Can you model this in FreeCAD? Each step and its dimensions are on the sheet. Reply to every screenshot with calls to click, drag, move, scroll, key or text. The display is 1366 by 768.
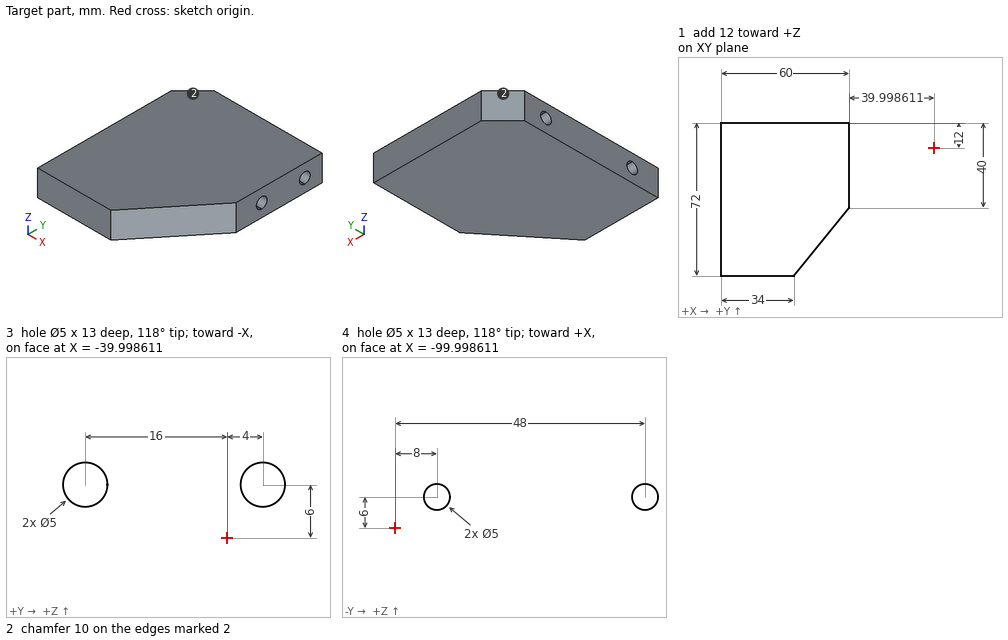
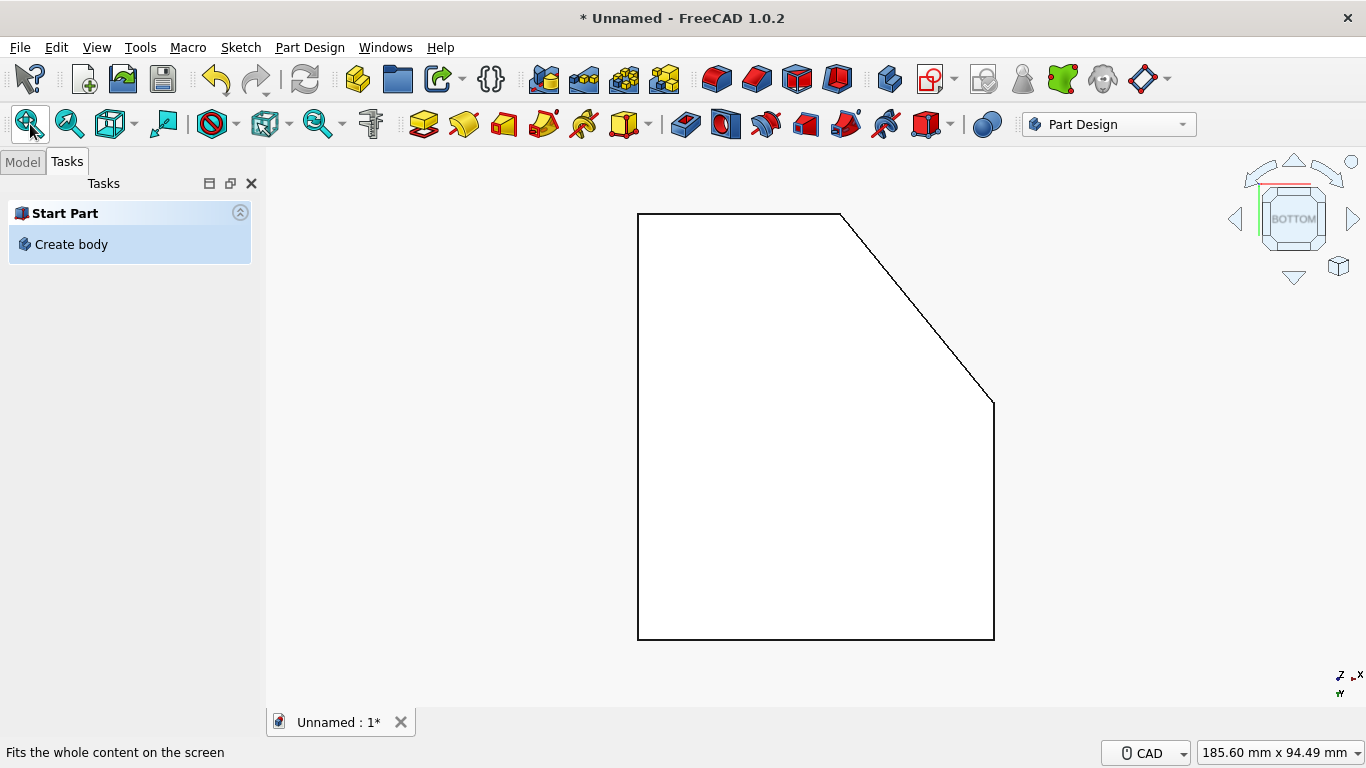
key(4)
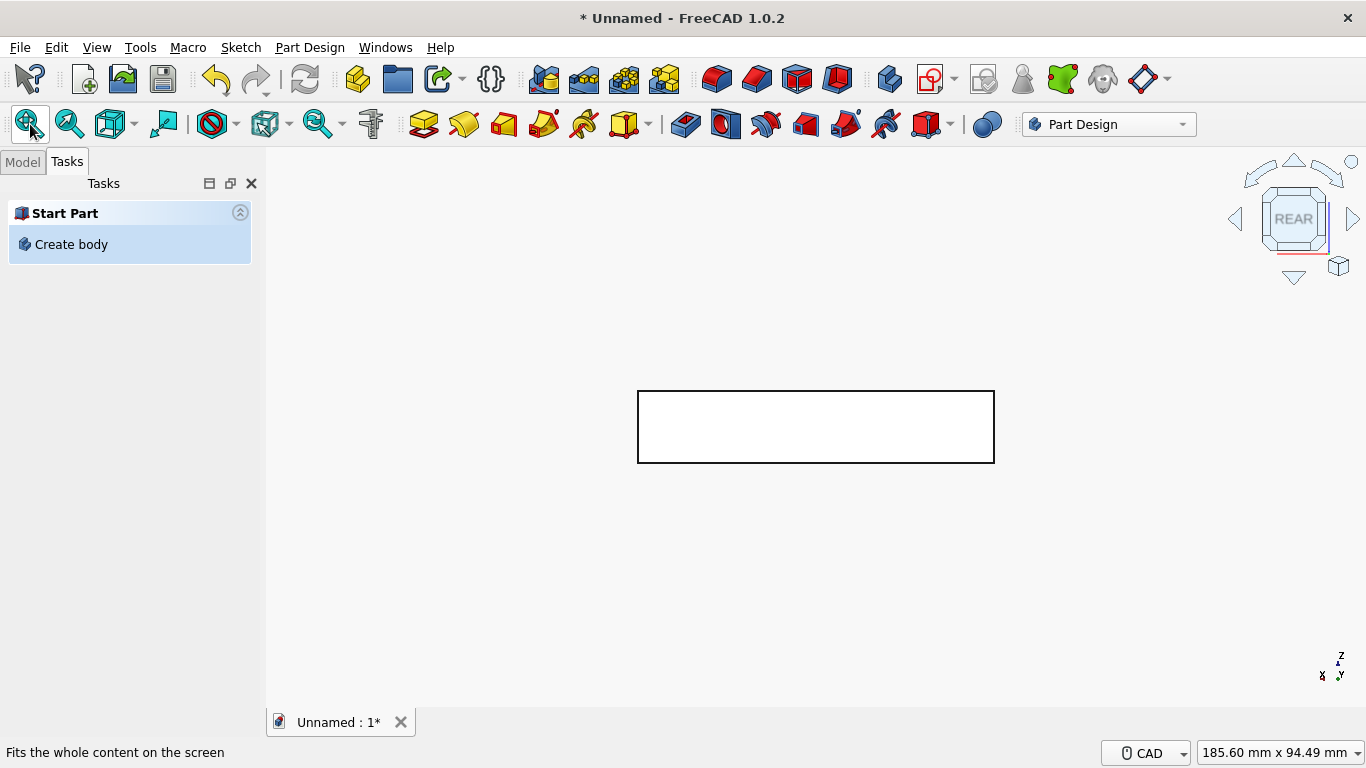
key(v)
key(f)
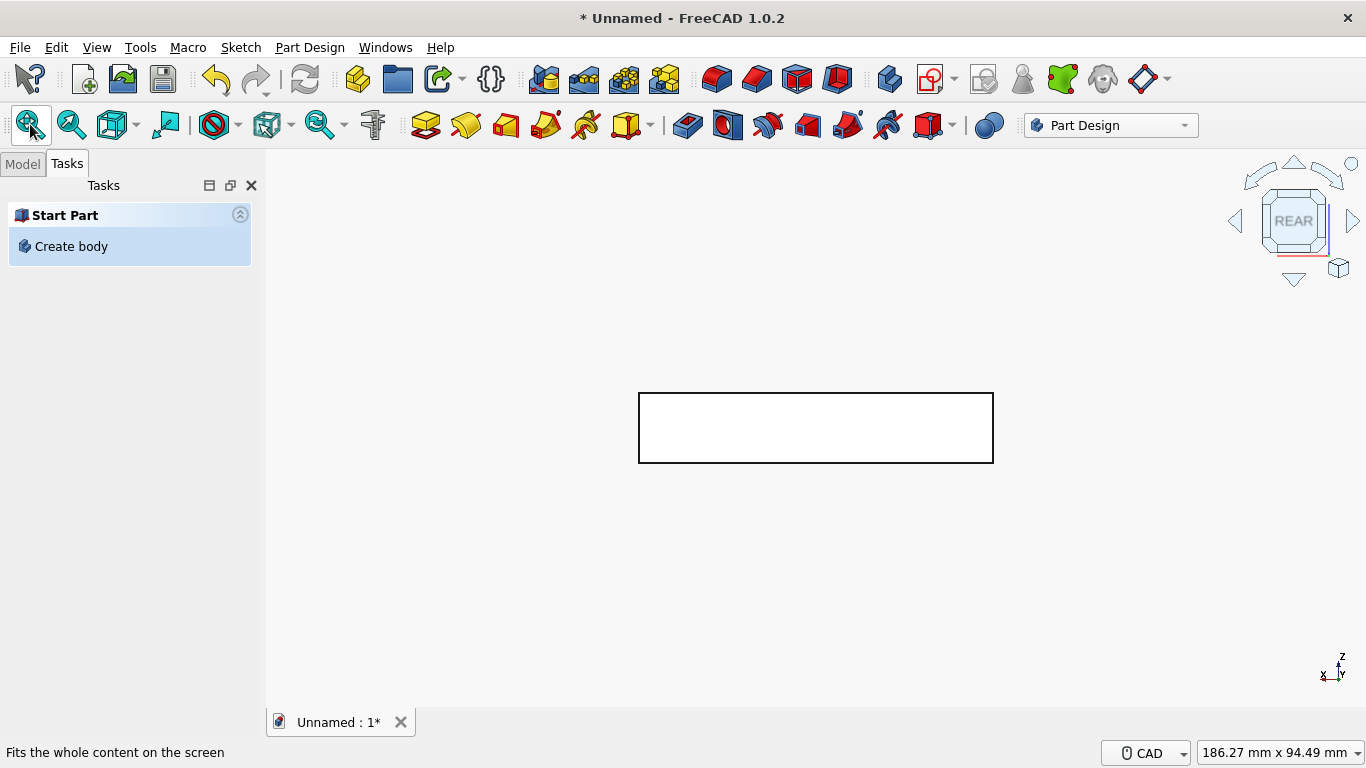
click(993, 427)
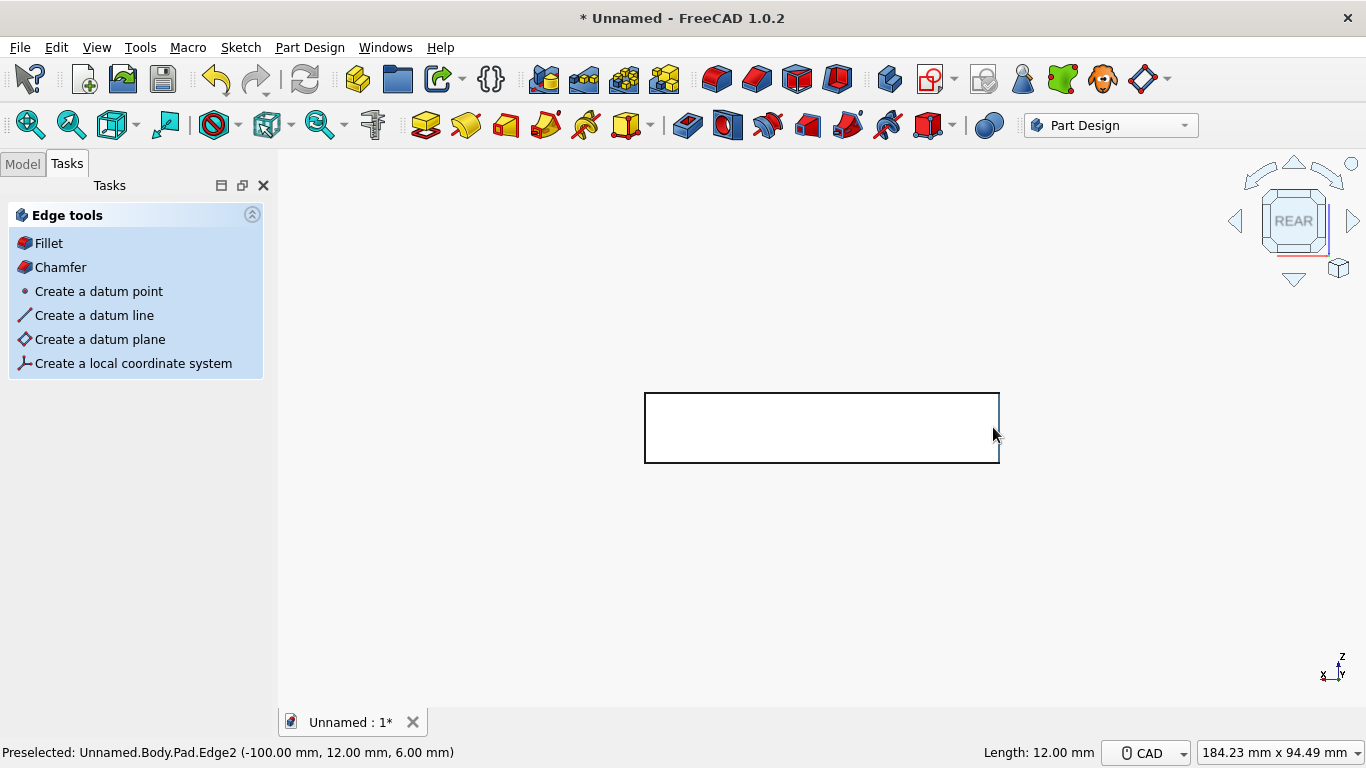
click(758, 80)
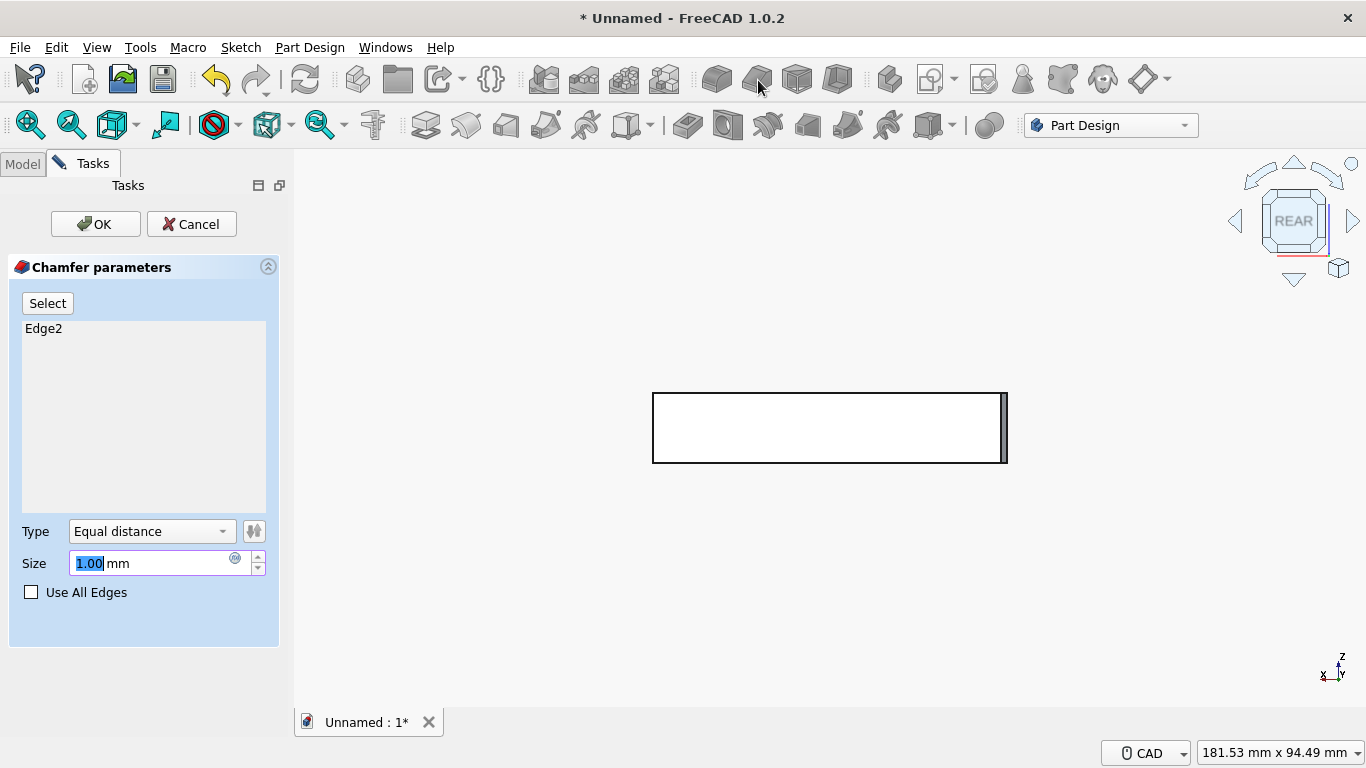
text(10)
key(Tab)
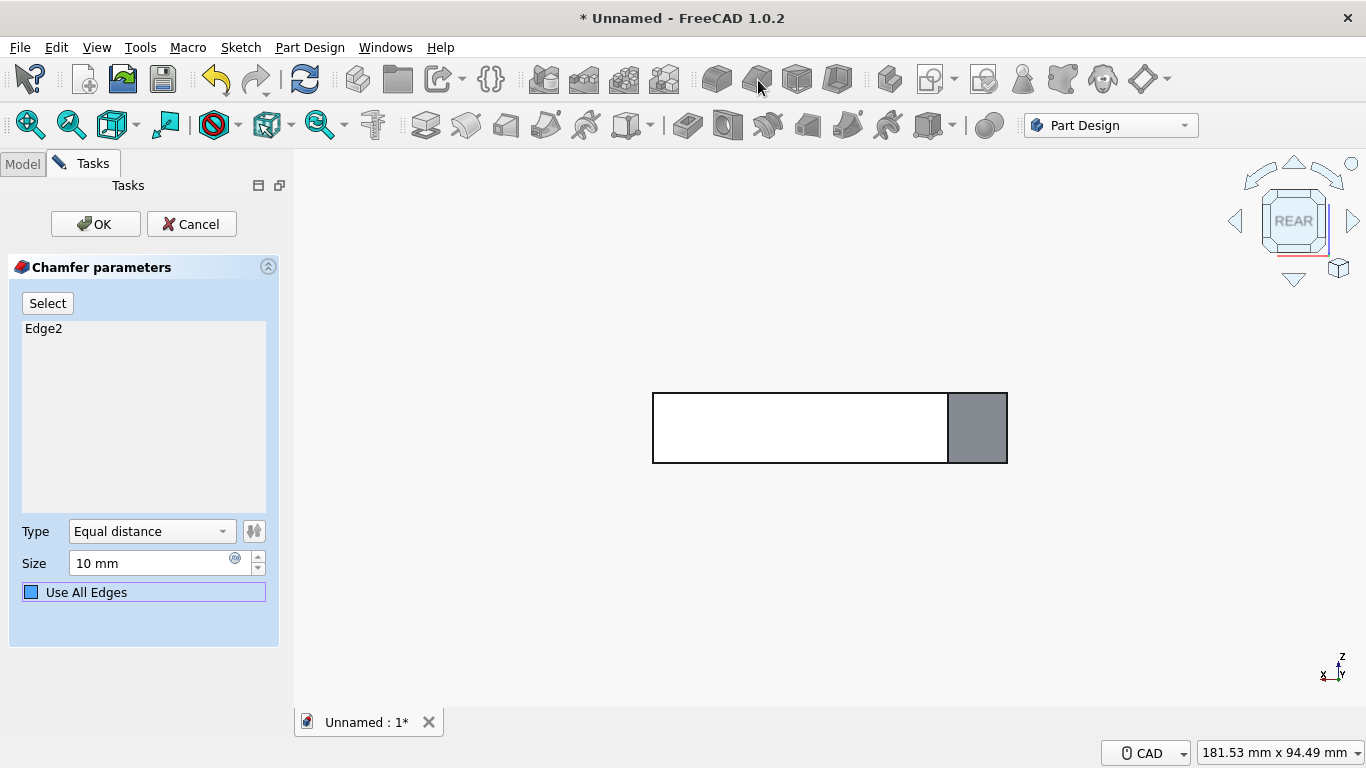
click(96, 224)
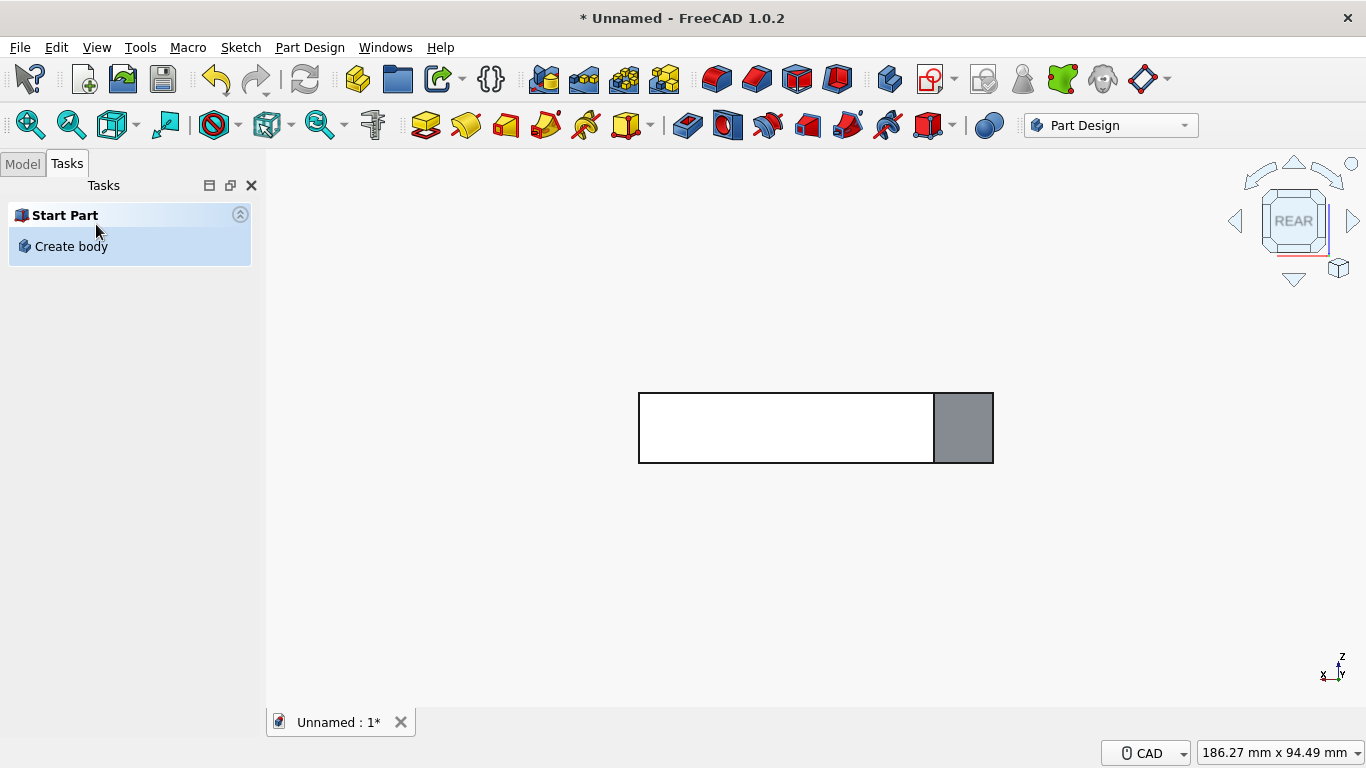
click(32, 126)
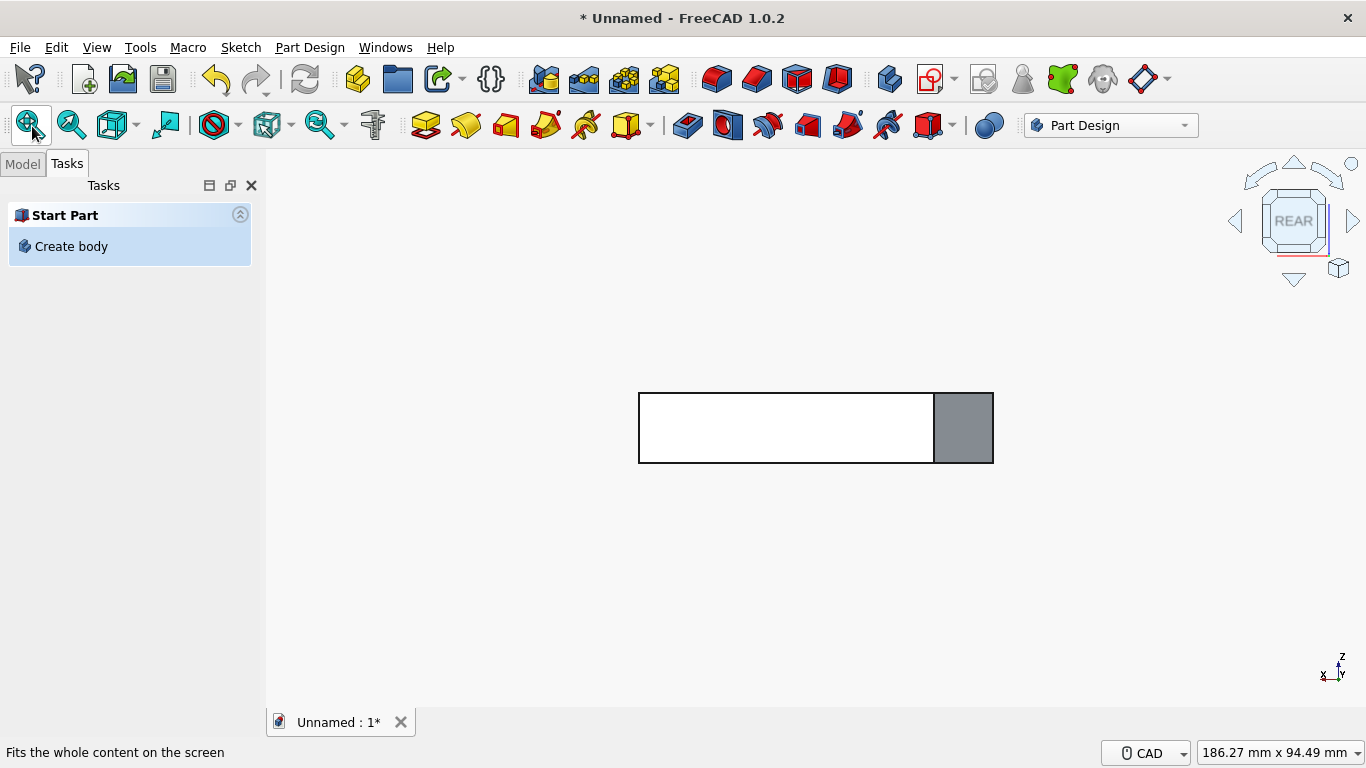
key(0)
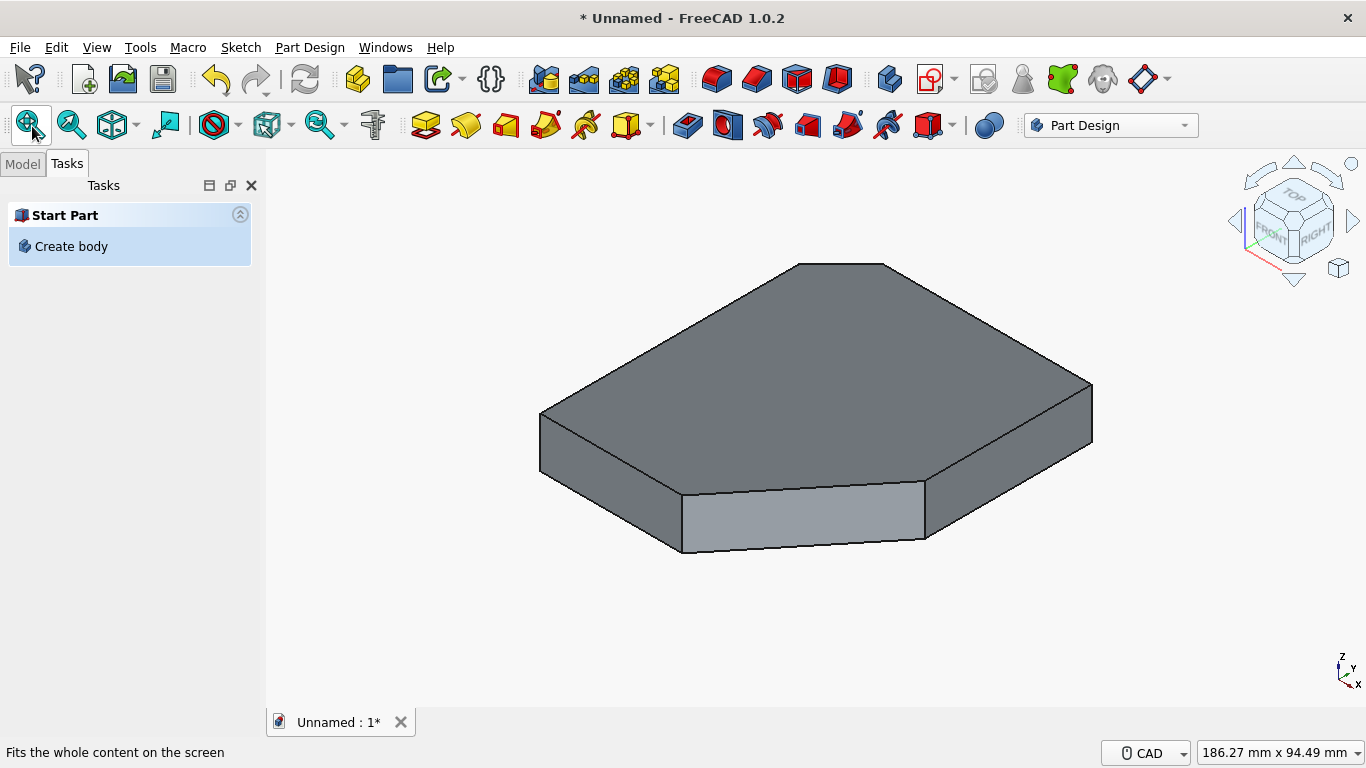
click(1056, 433)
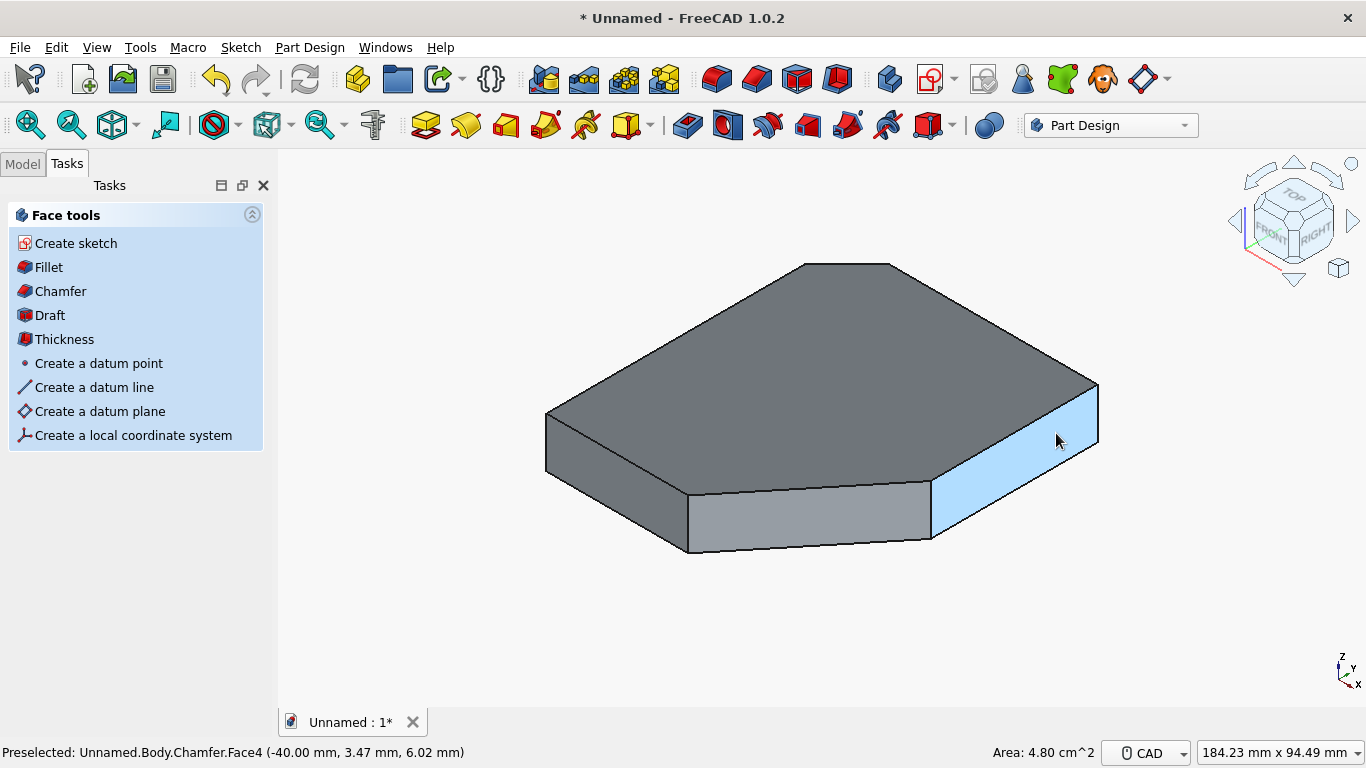
click(930, 80)